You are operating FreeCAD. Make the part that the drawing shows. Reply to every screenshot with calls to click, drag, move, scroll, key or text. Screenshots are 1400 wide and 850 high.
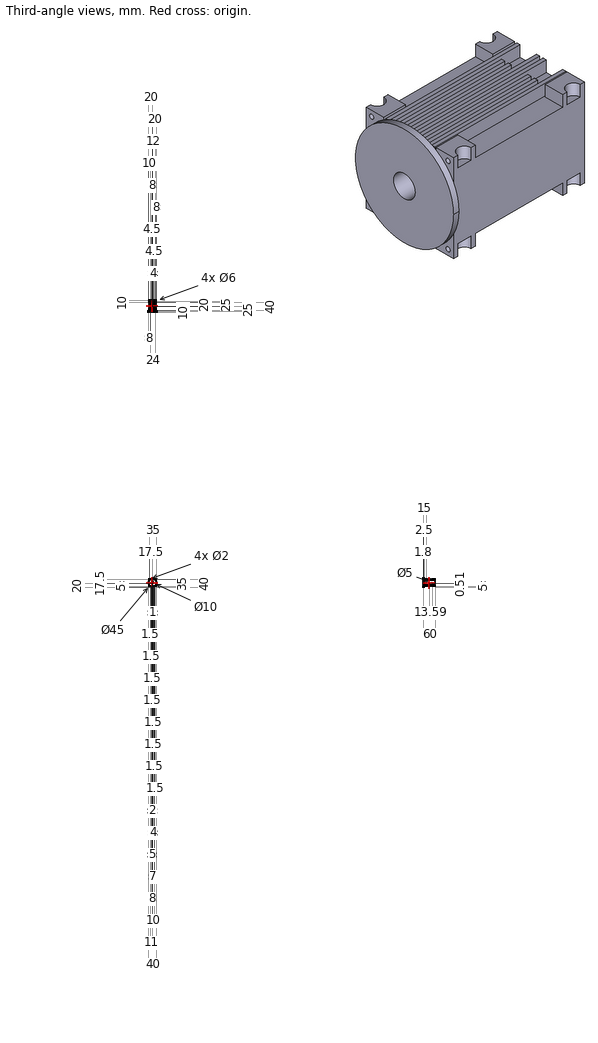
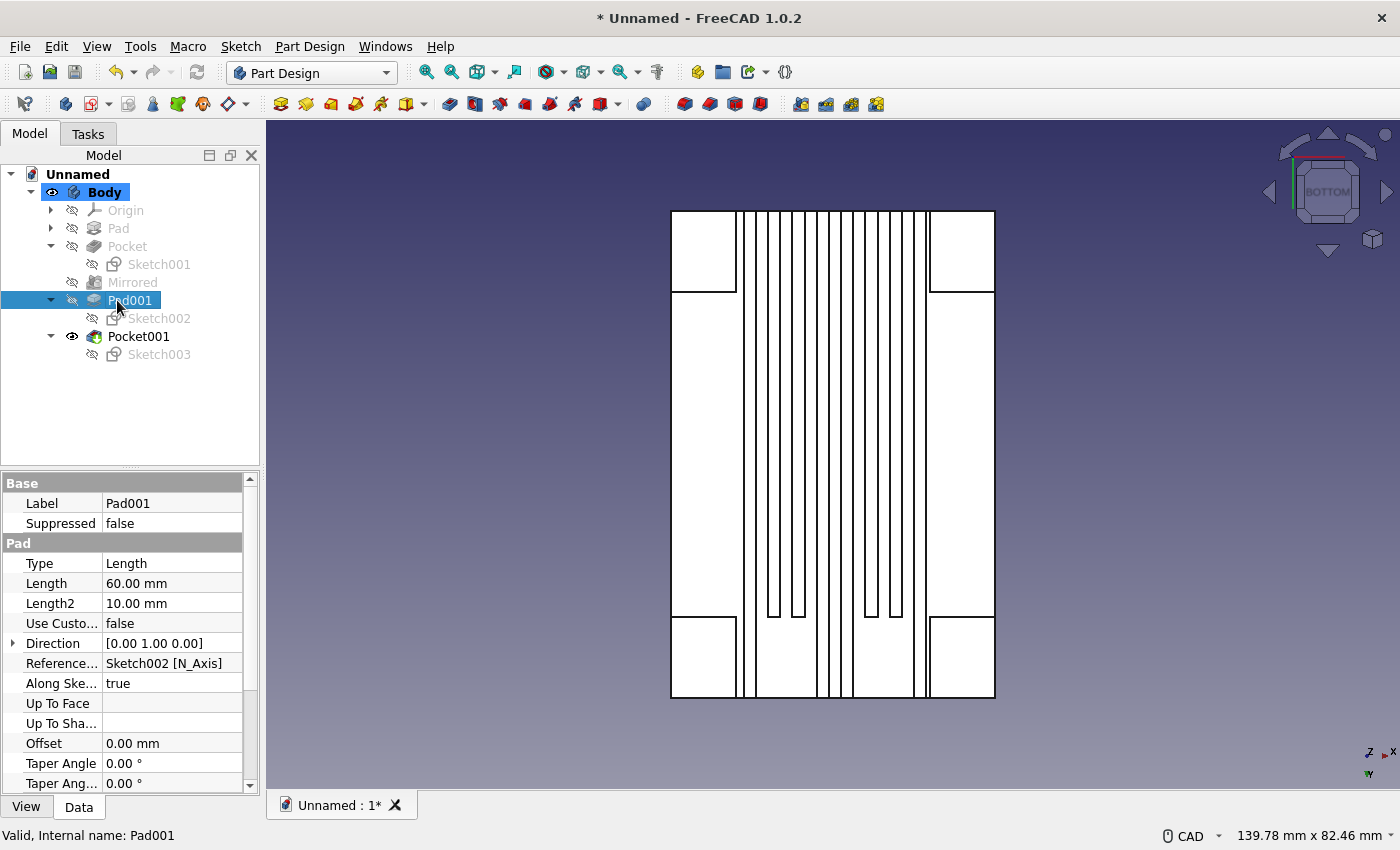
click(117, 336, ctrl)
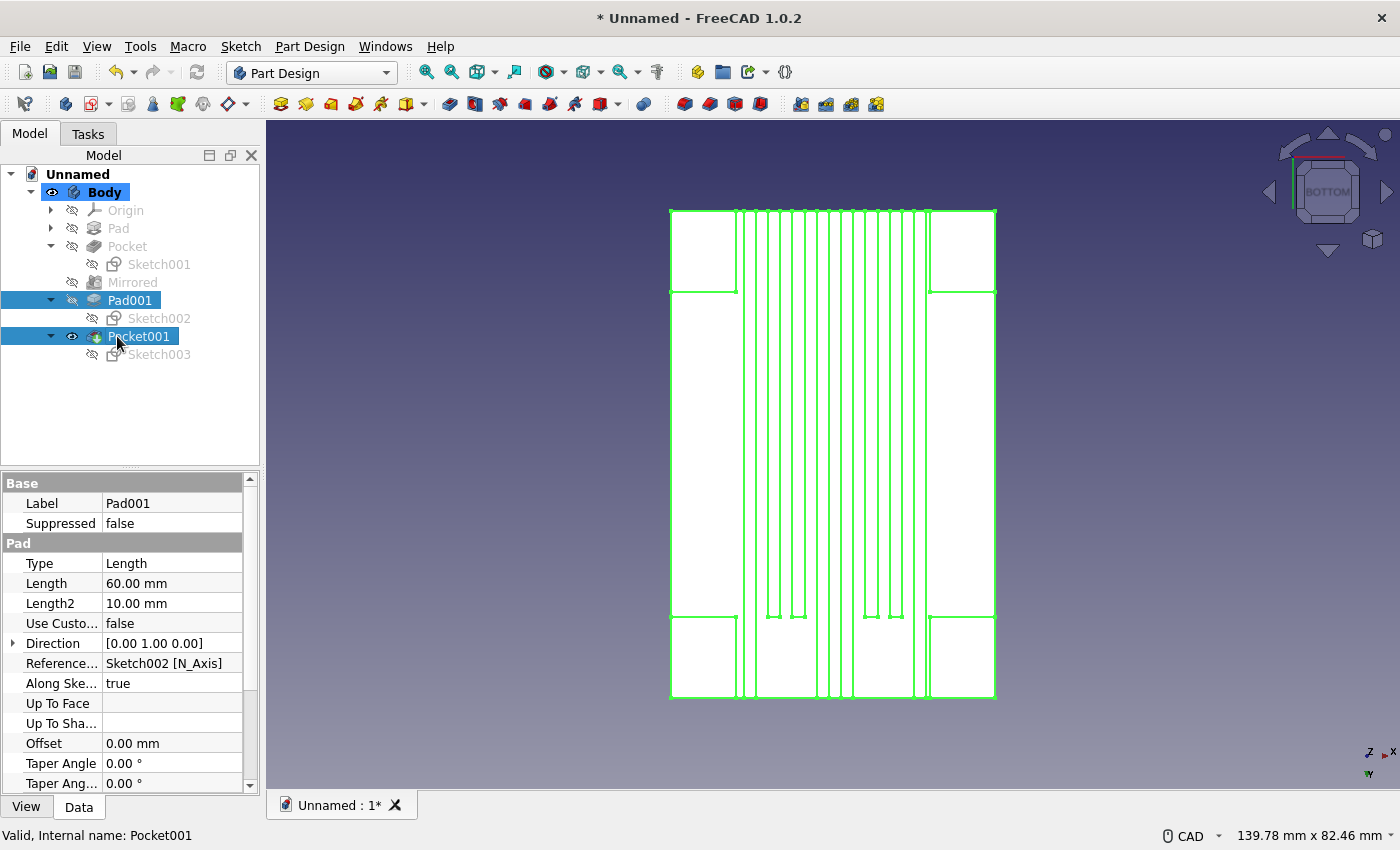
click(801, 104)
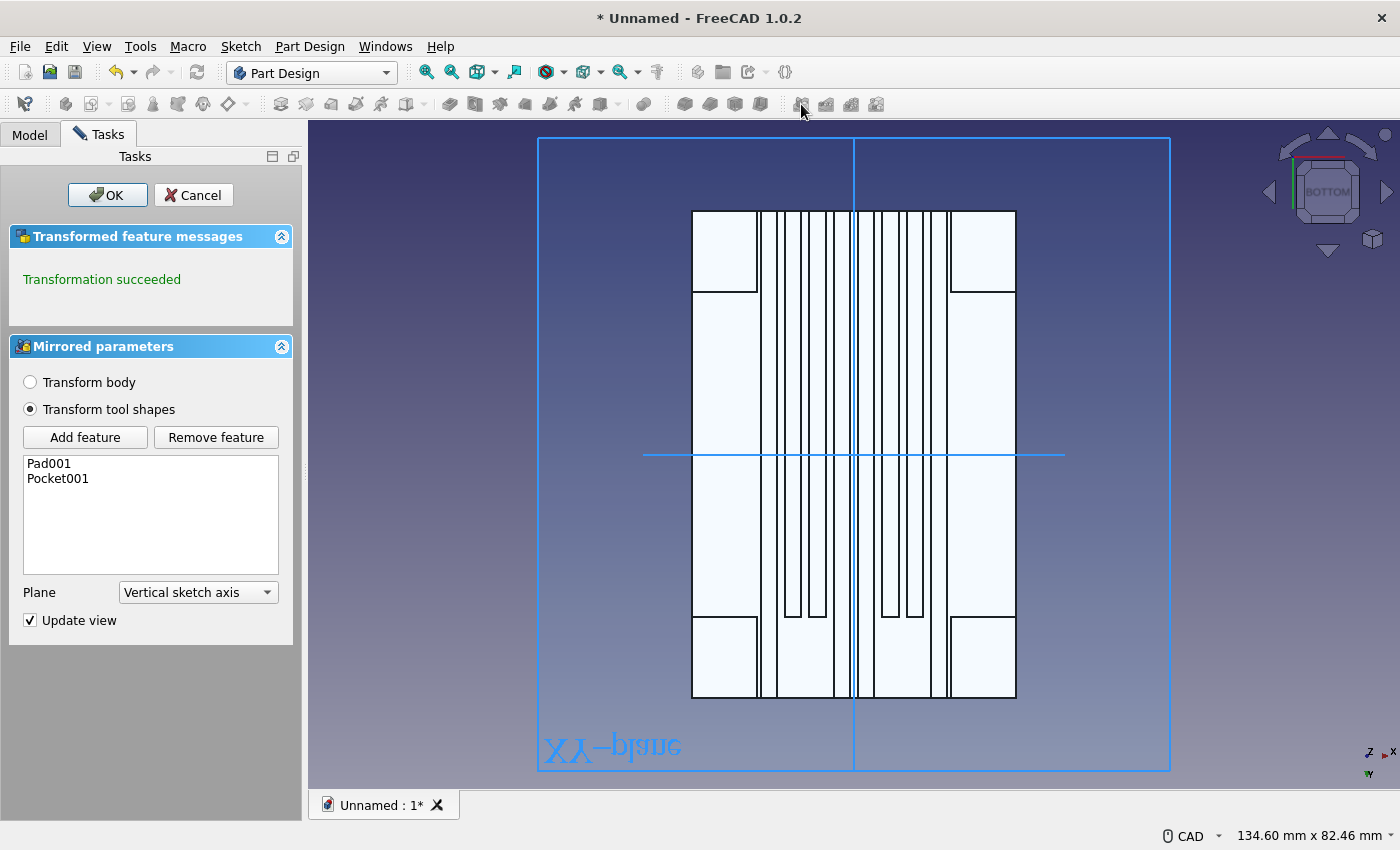
click(199, 592)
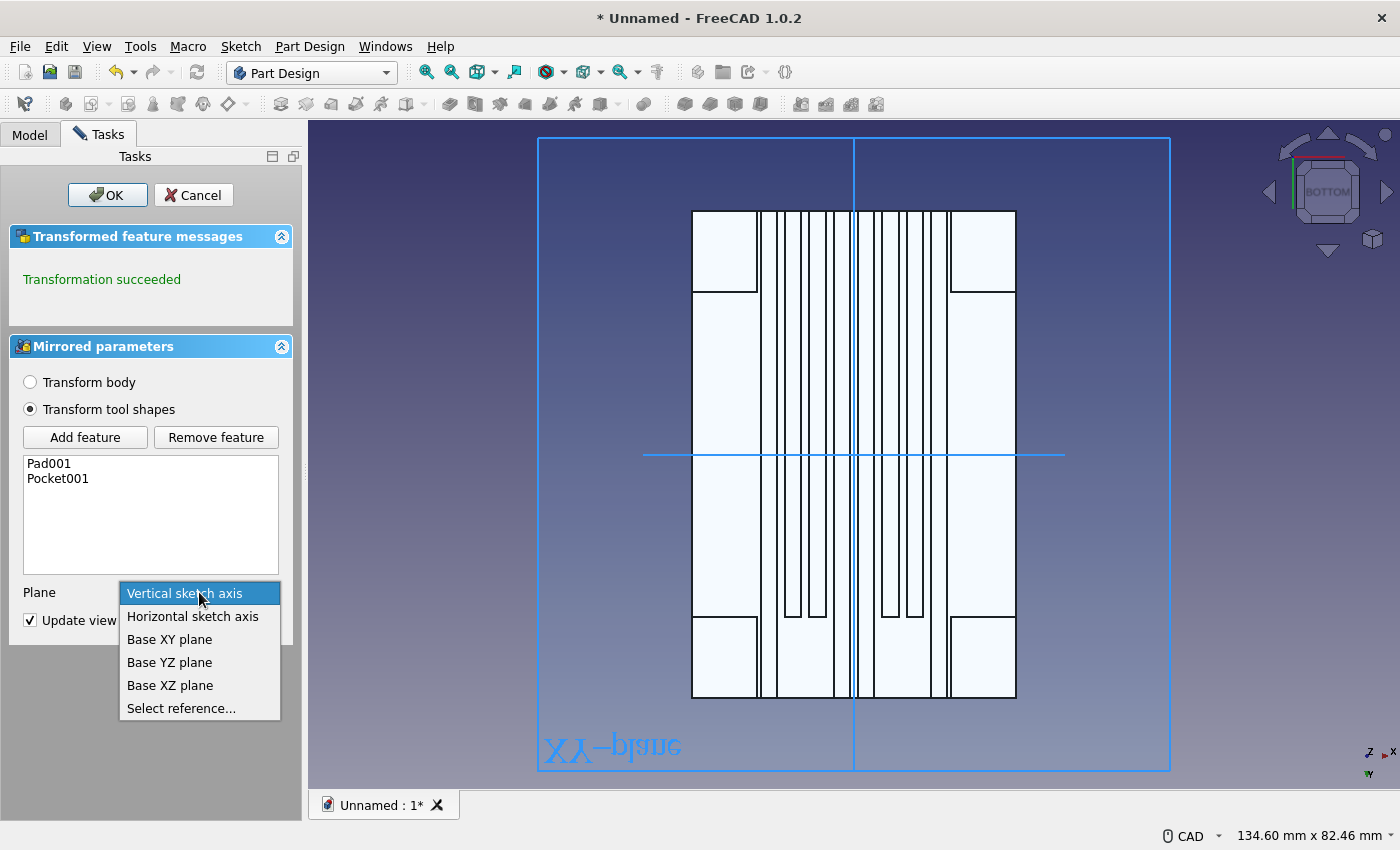
click(198, 640)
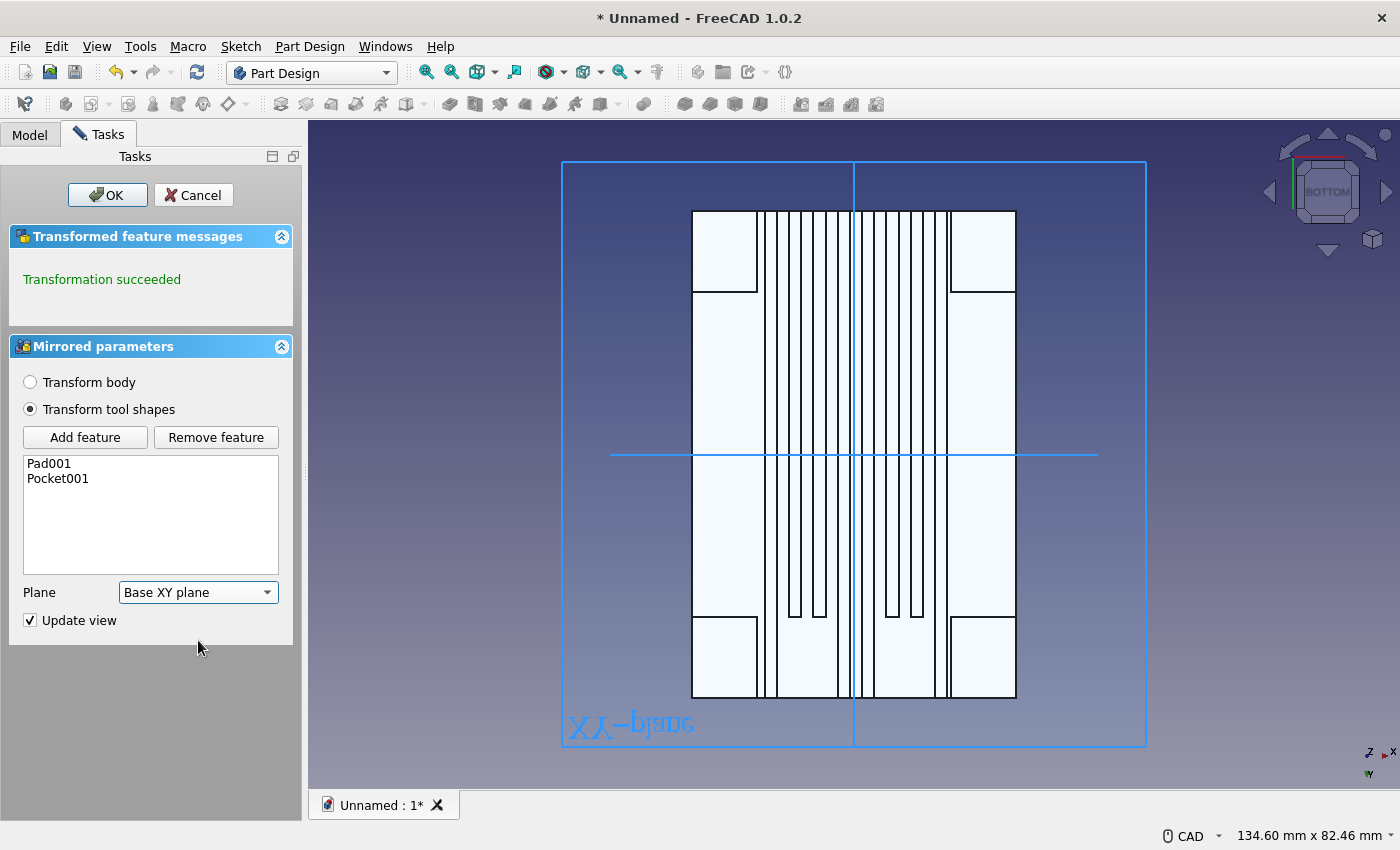
click(108, 195)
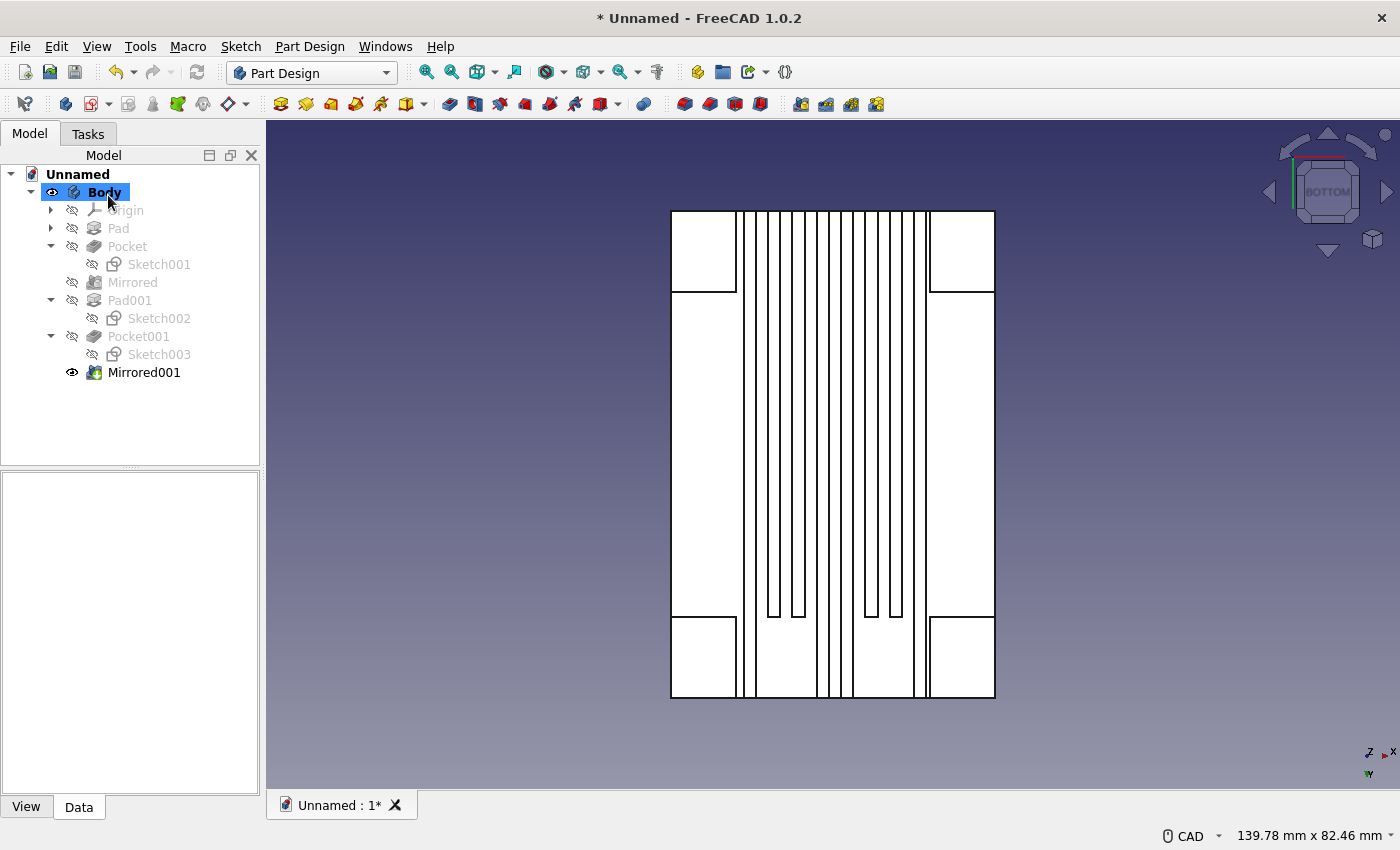
scroll(920, 662, up, 4)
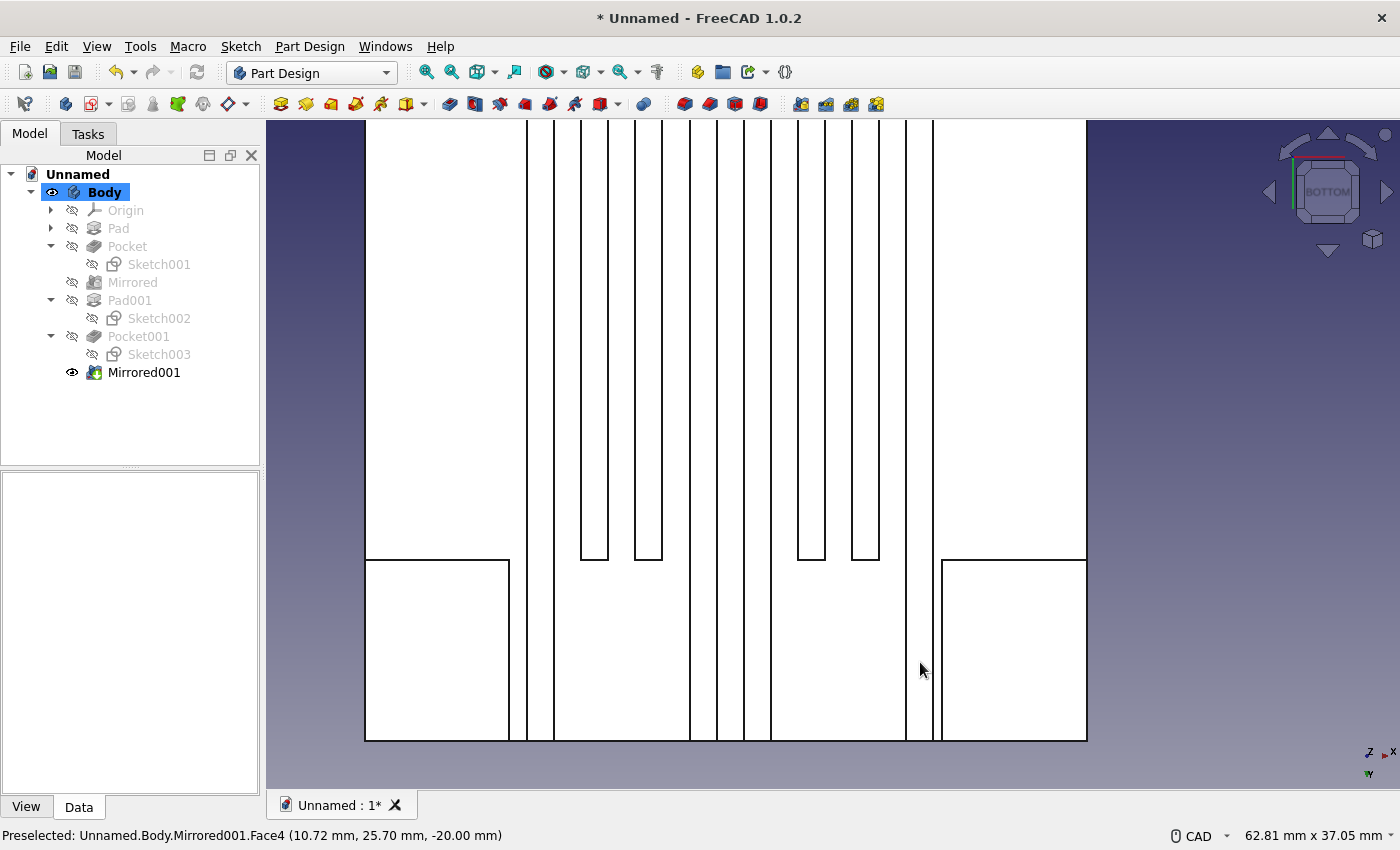
click(920, 662)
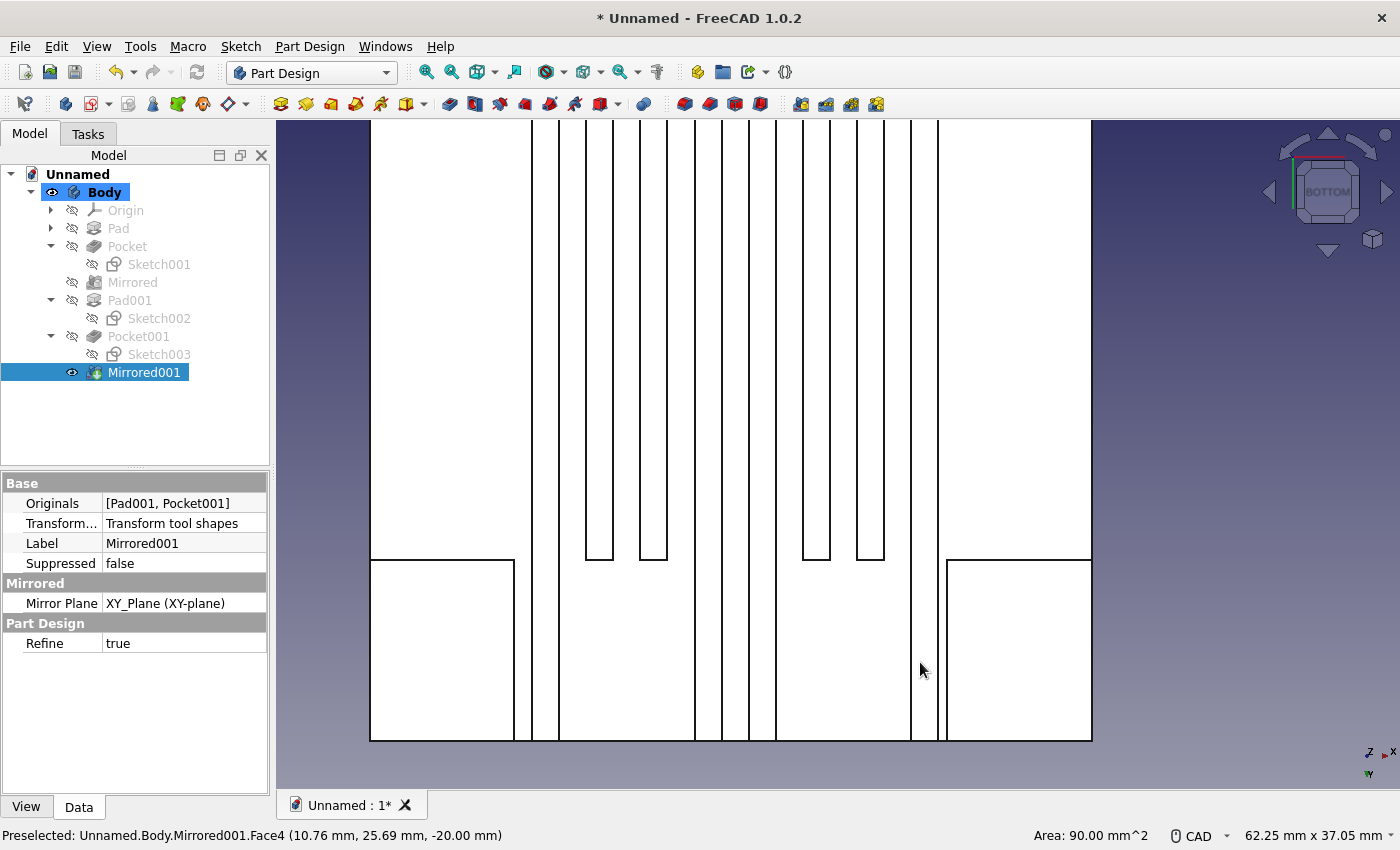
click(90, 104)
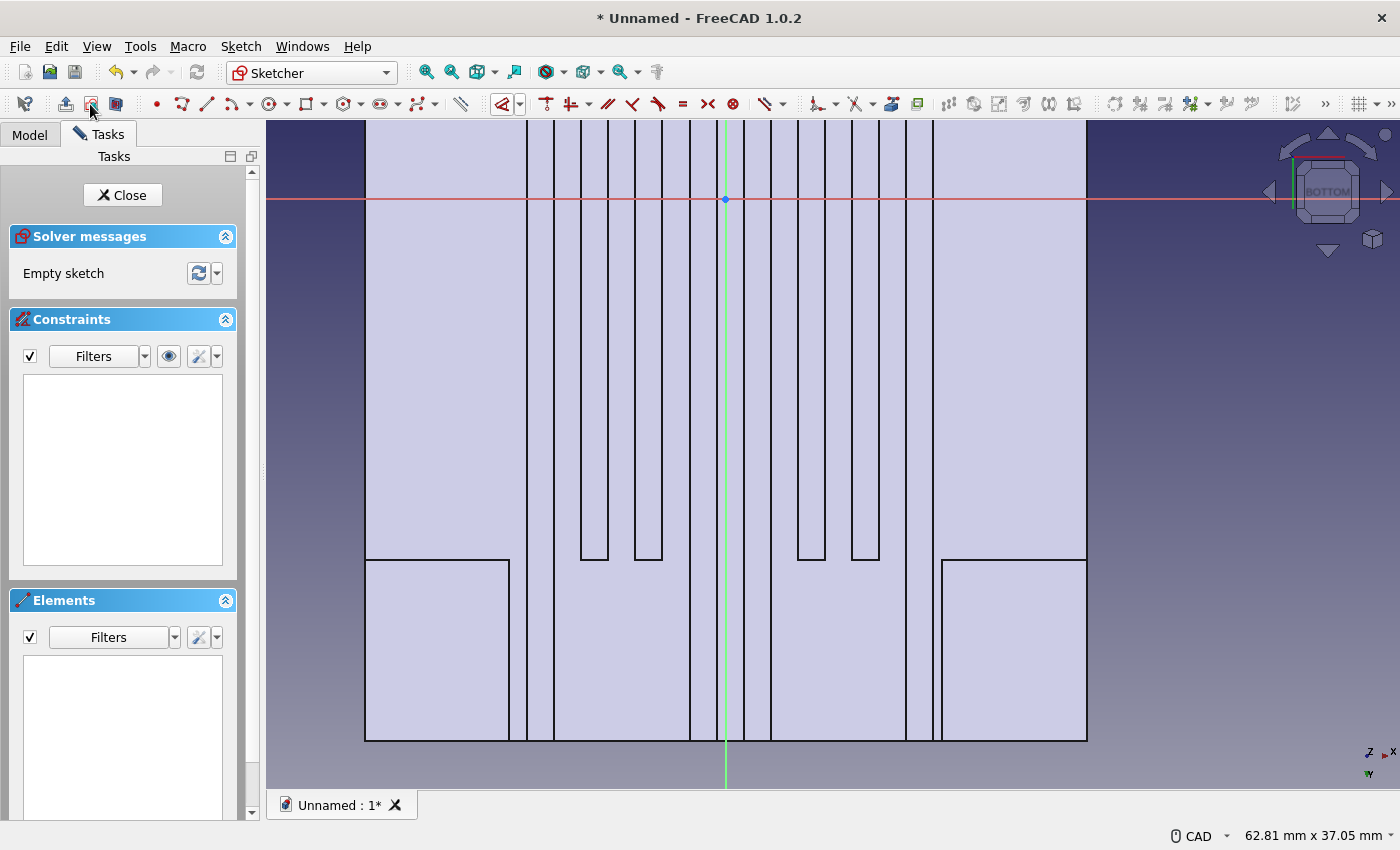
scroll(796, 663, down, 4)